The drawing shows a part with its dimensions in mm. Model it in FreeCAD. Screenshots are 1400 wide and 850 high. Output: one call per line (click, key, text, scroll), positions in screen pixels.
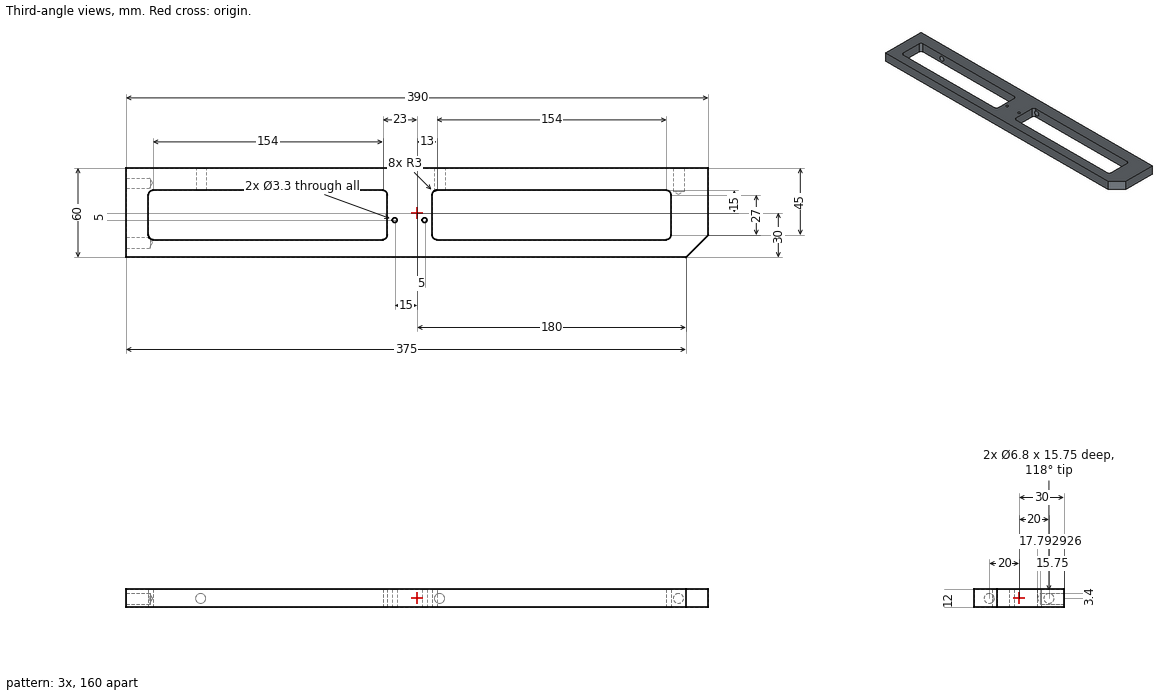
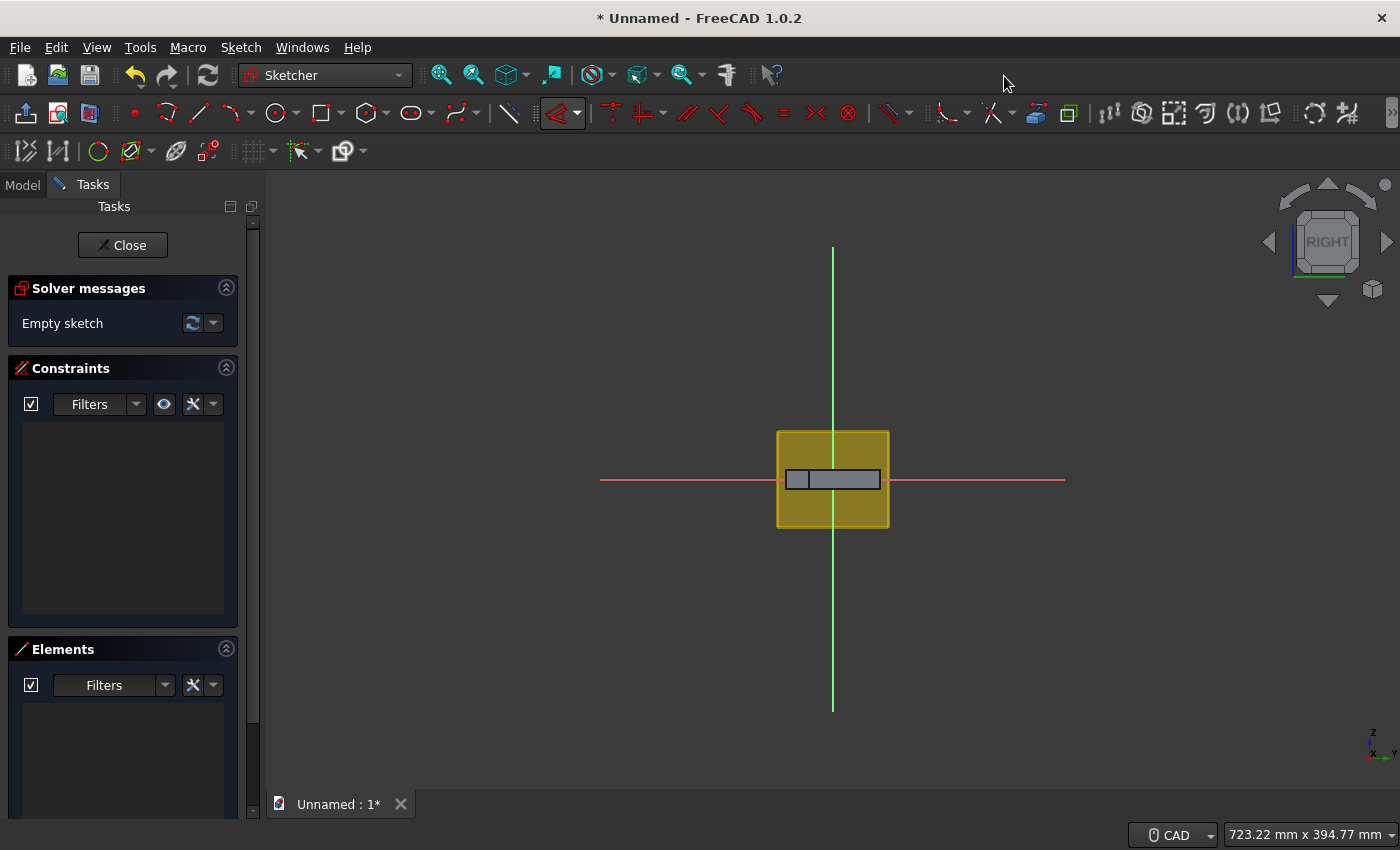
key(q)
key(s)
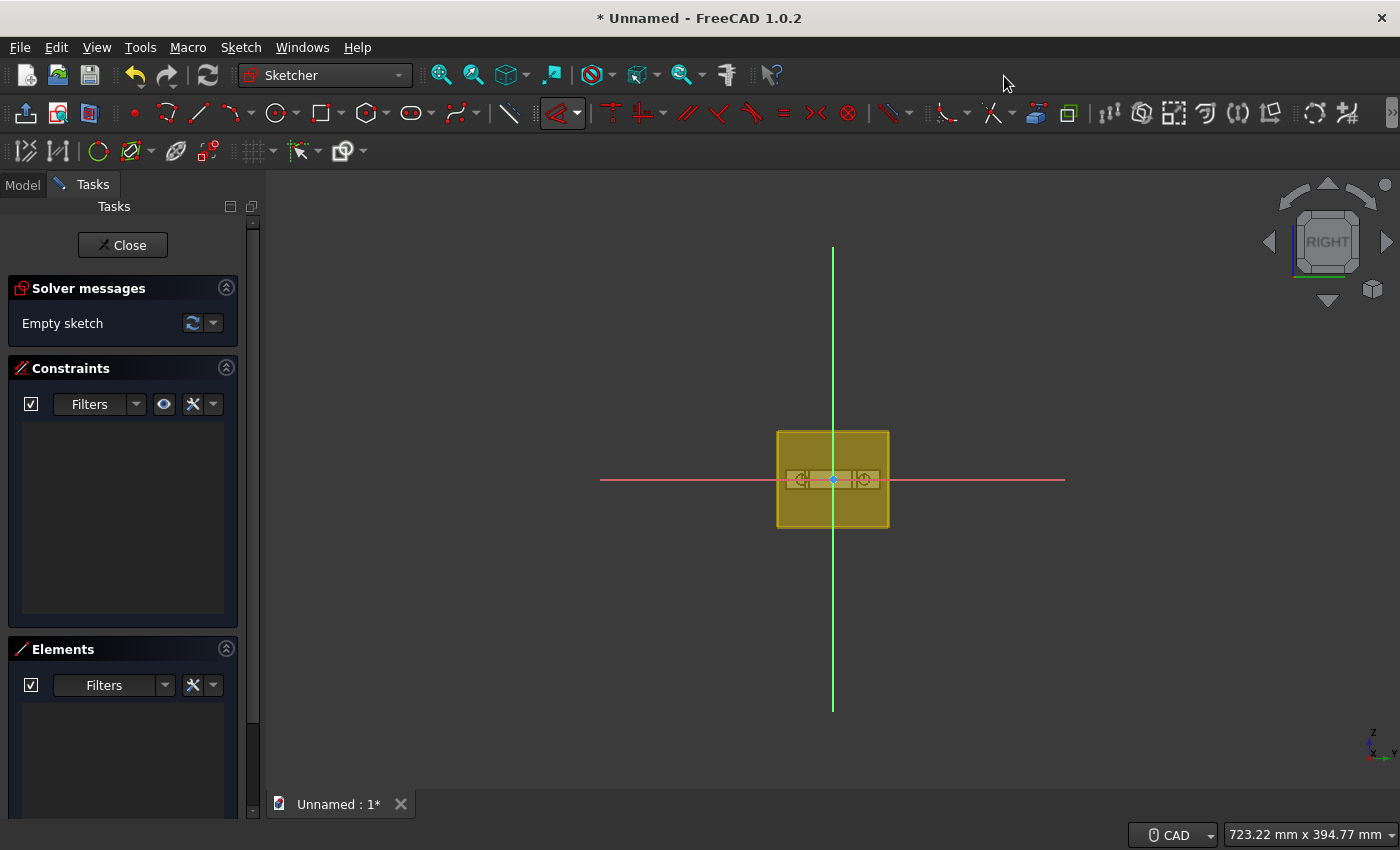
scroll(864, 477, up, 13)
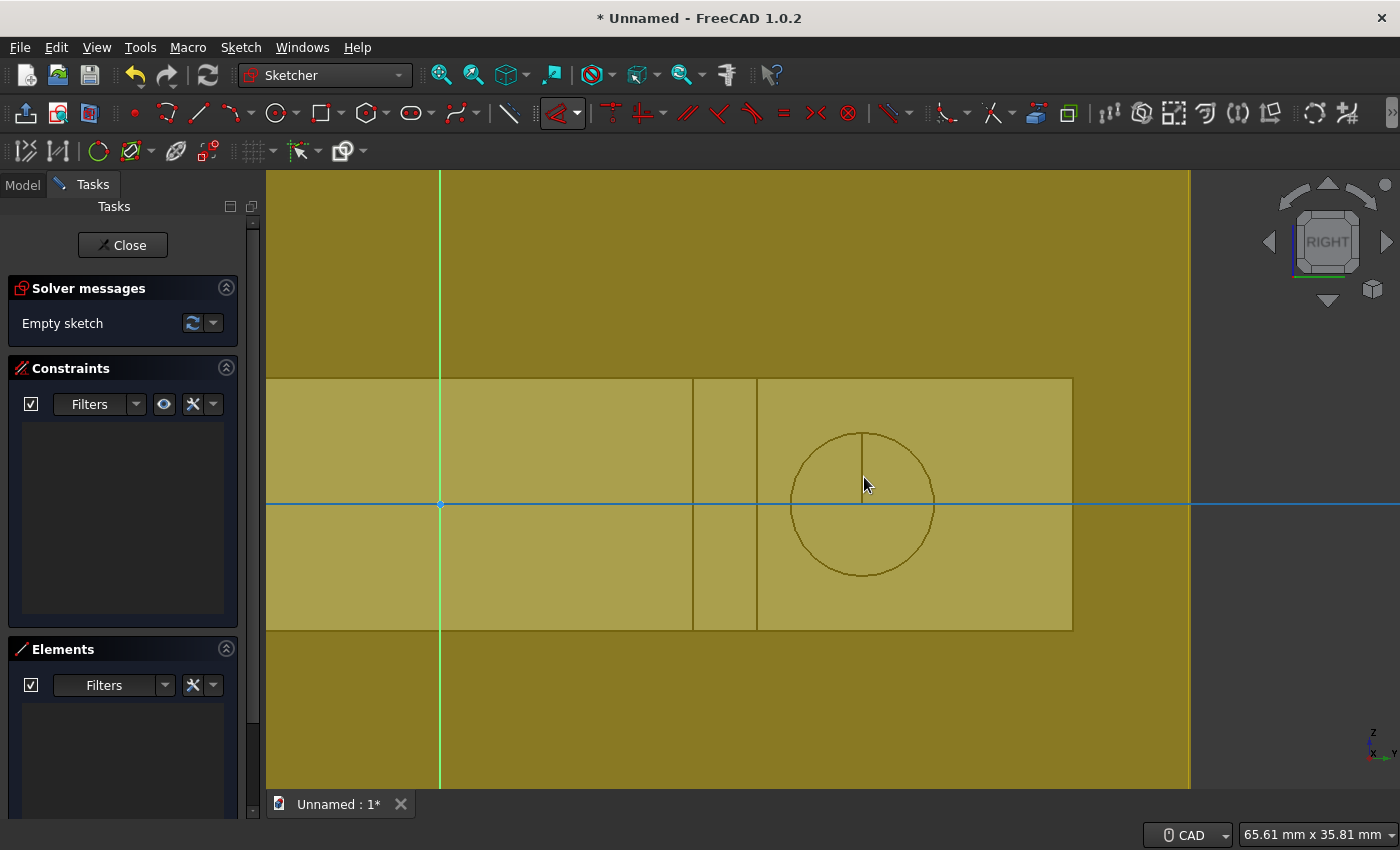
key(g)
key(m)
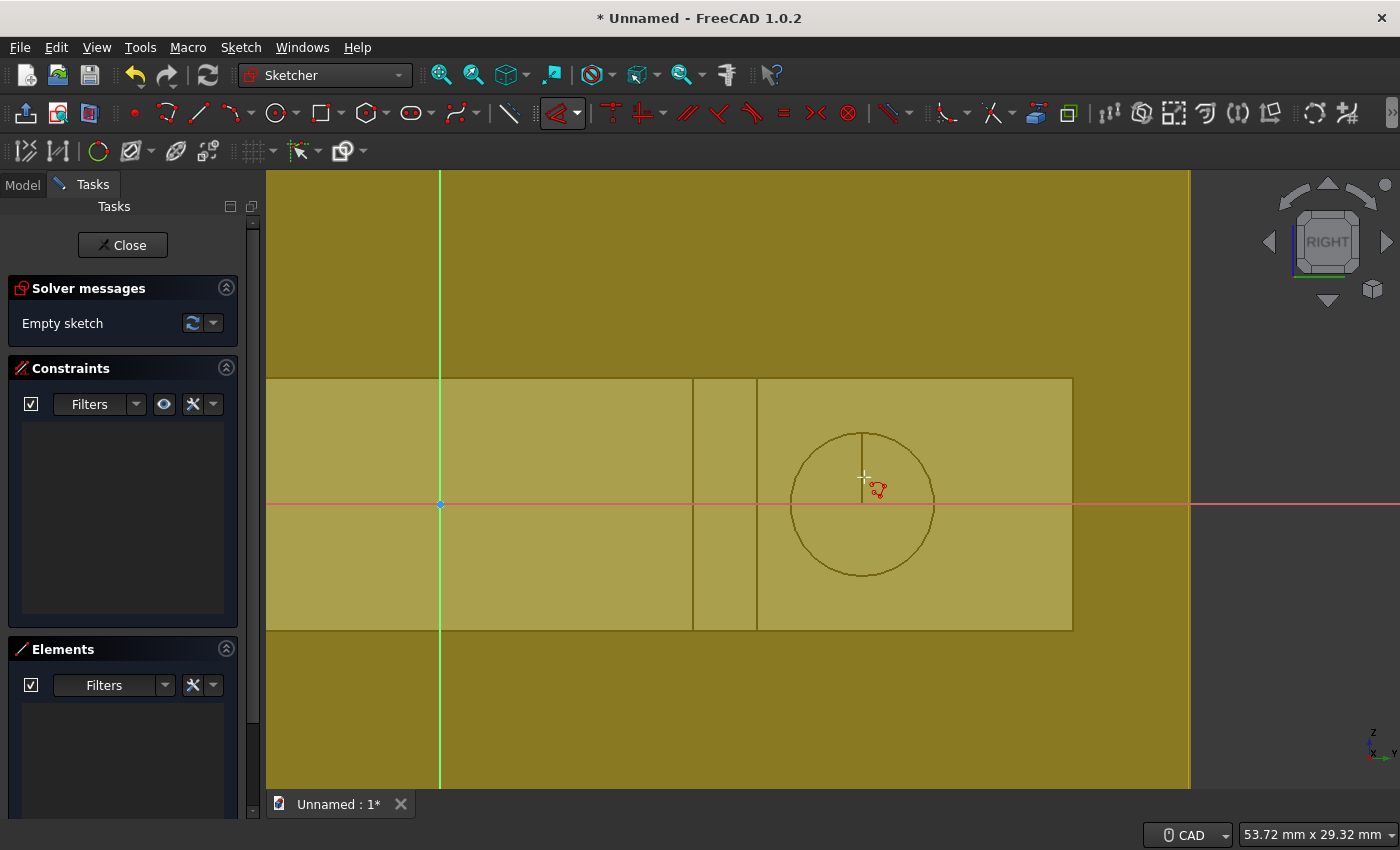
click(698, 504)
click(1073, 495)
click(1073, 433)
click(741, 433)
click(698, 504)
key(Escape)
key(Escape)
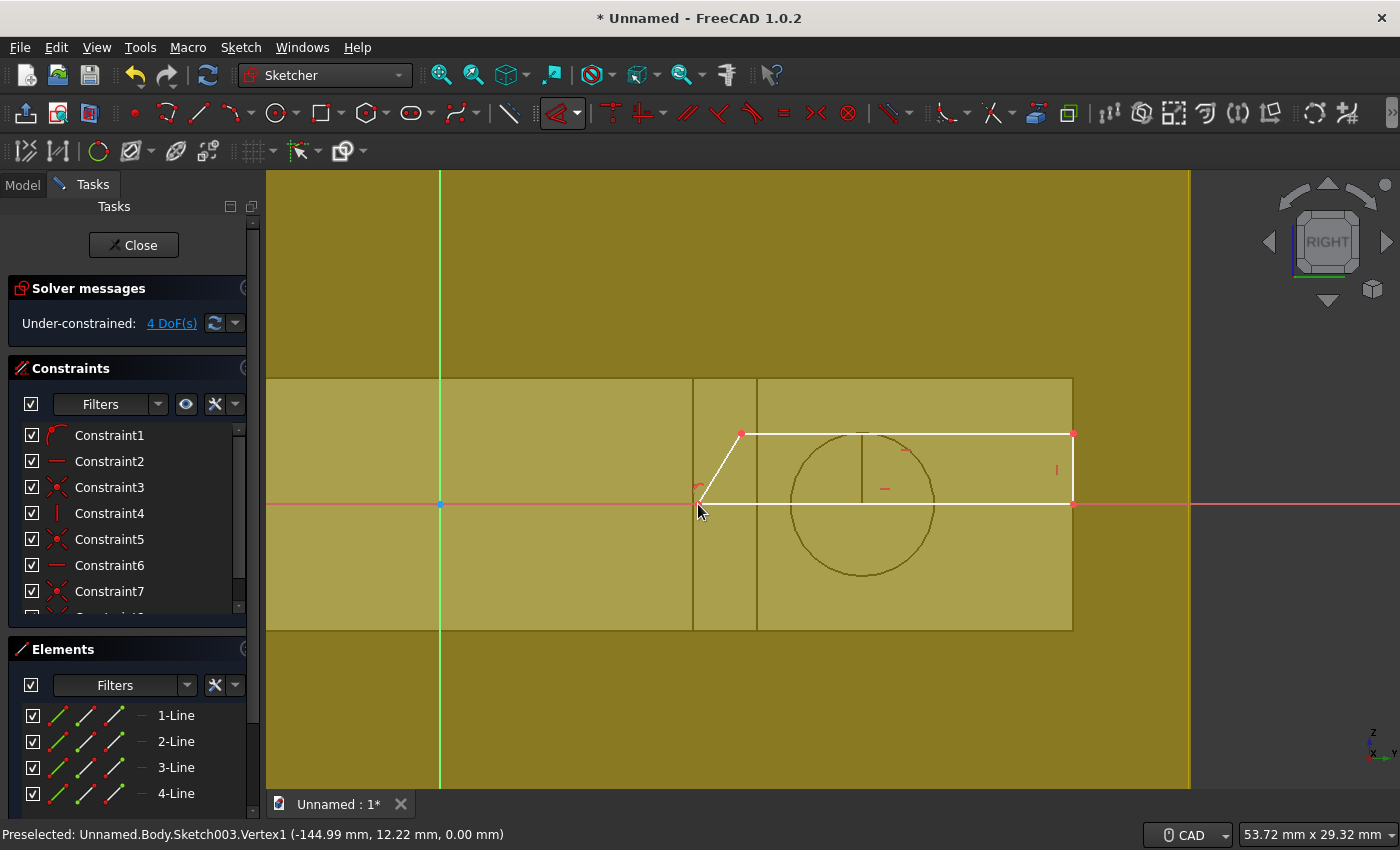
click(1073, 483)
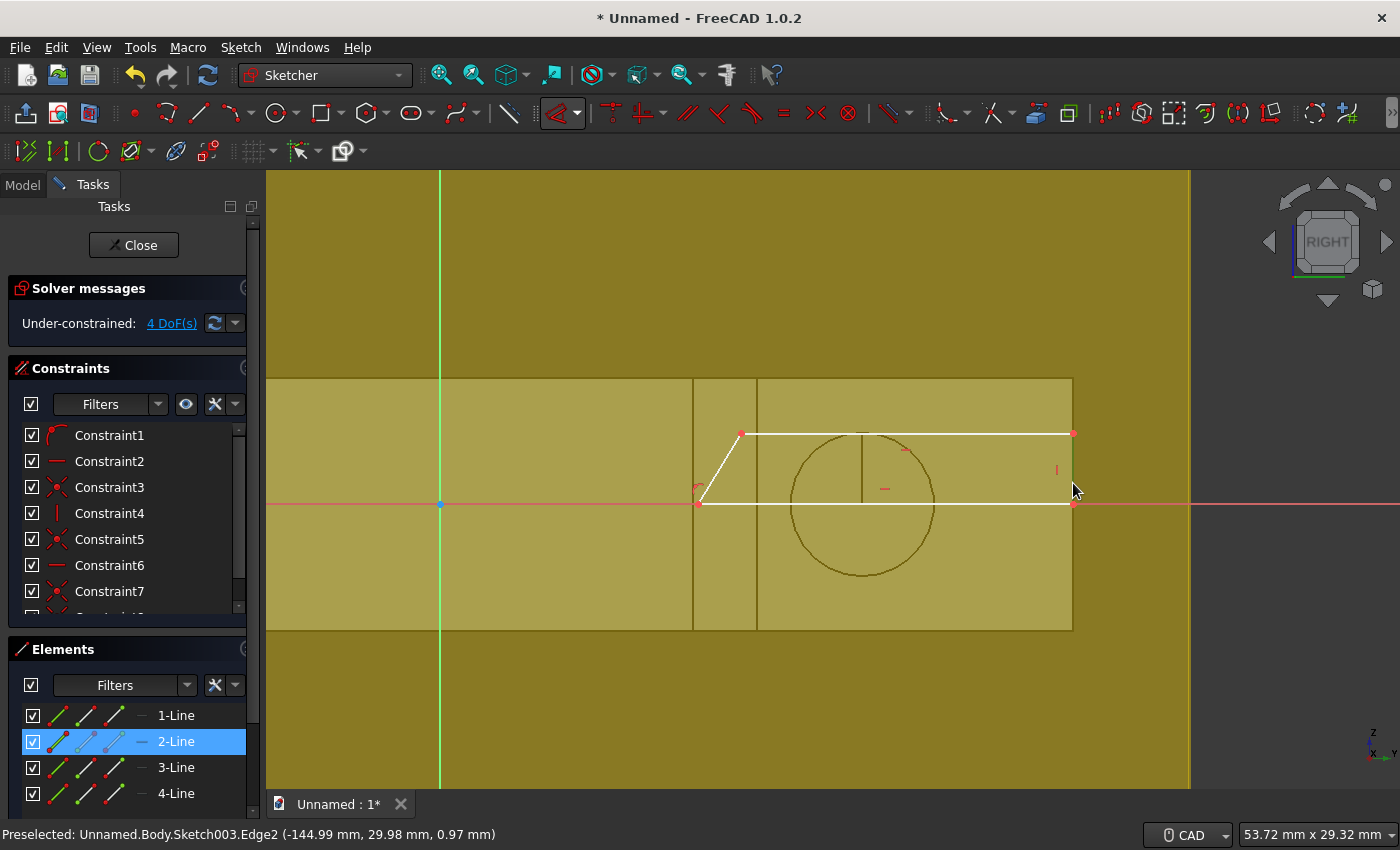
key(i)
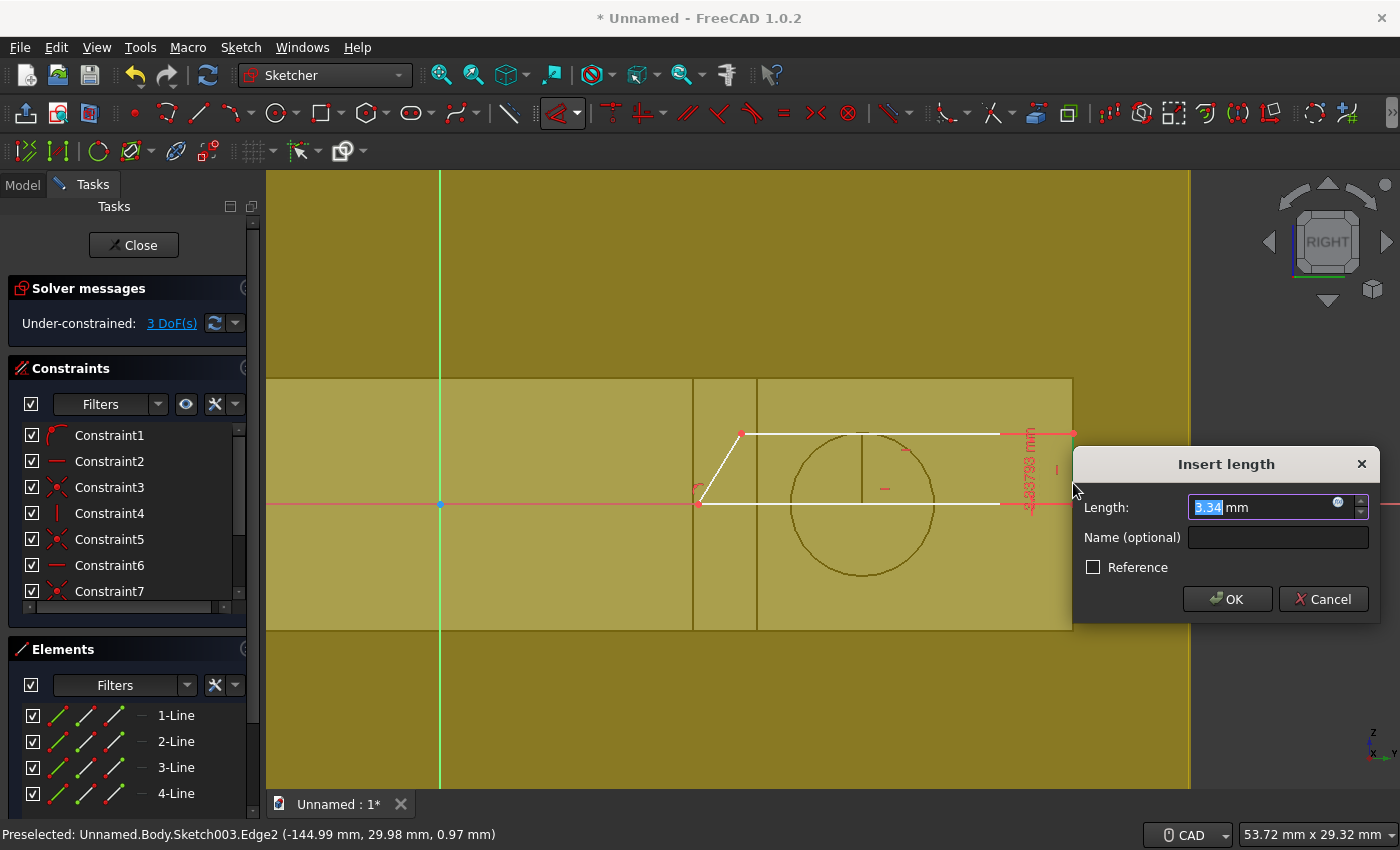
text(3.4)
key(Return)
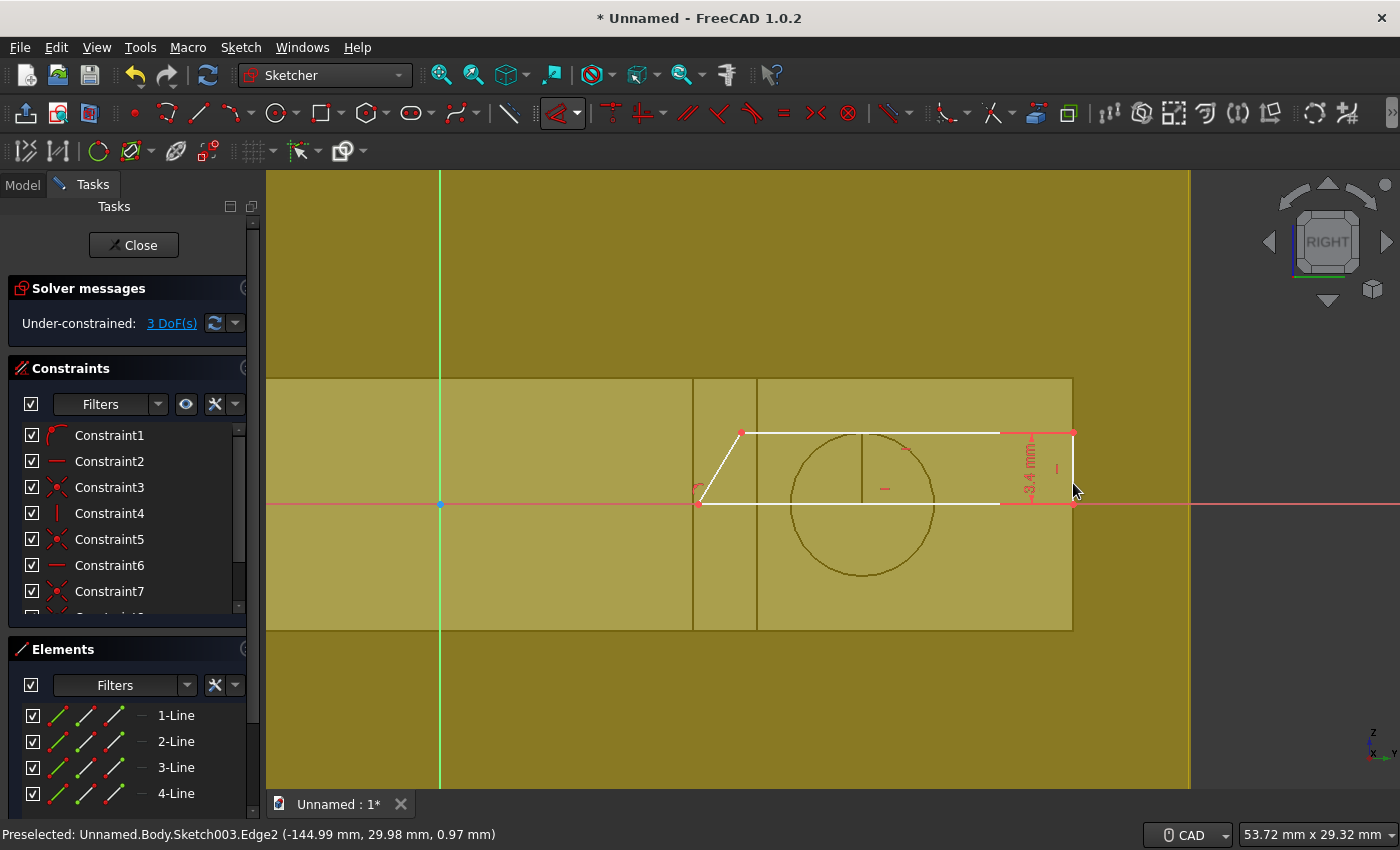
click(1073, 504)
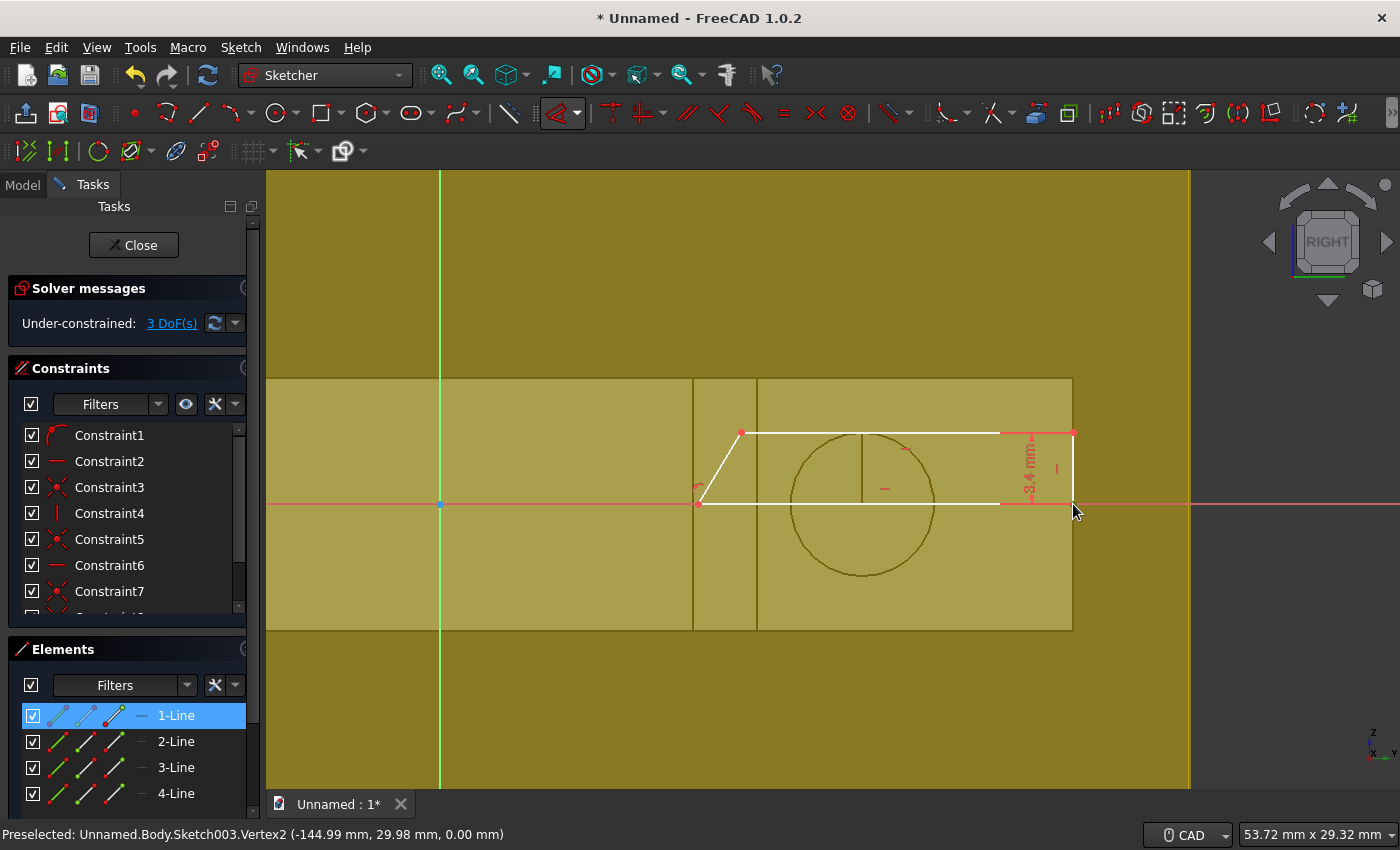
key(l)